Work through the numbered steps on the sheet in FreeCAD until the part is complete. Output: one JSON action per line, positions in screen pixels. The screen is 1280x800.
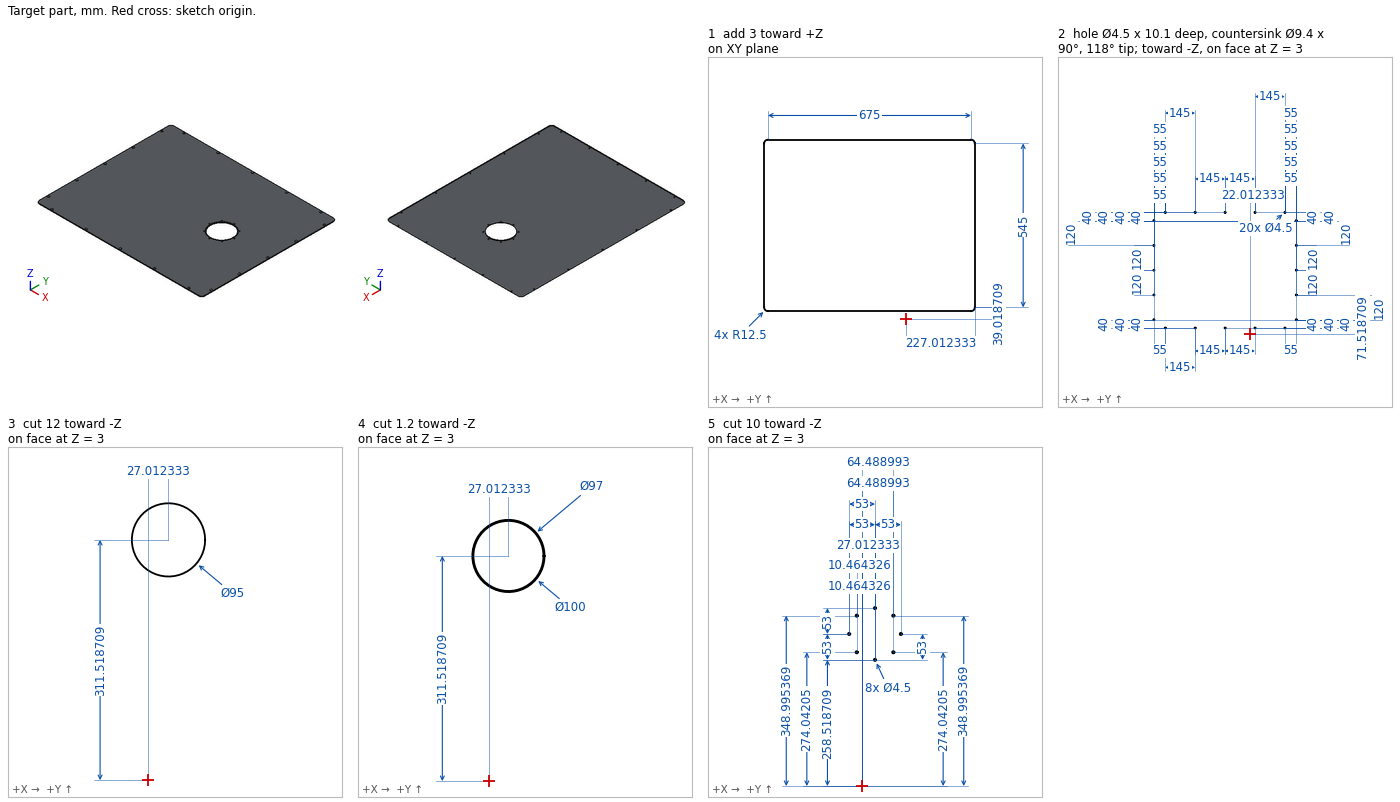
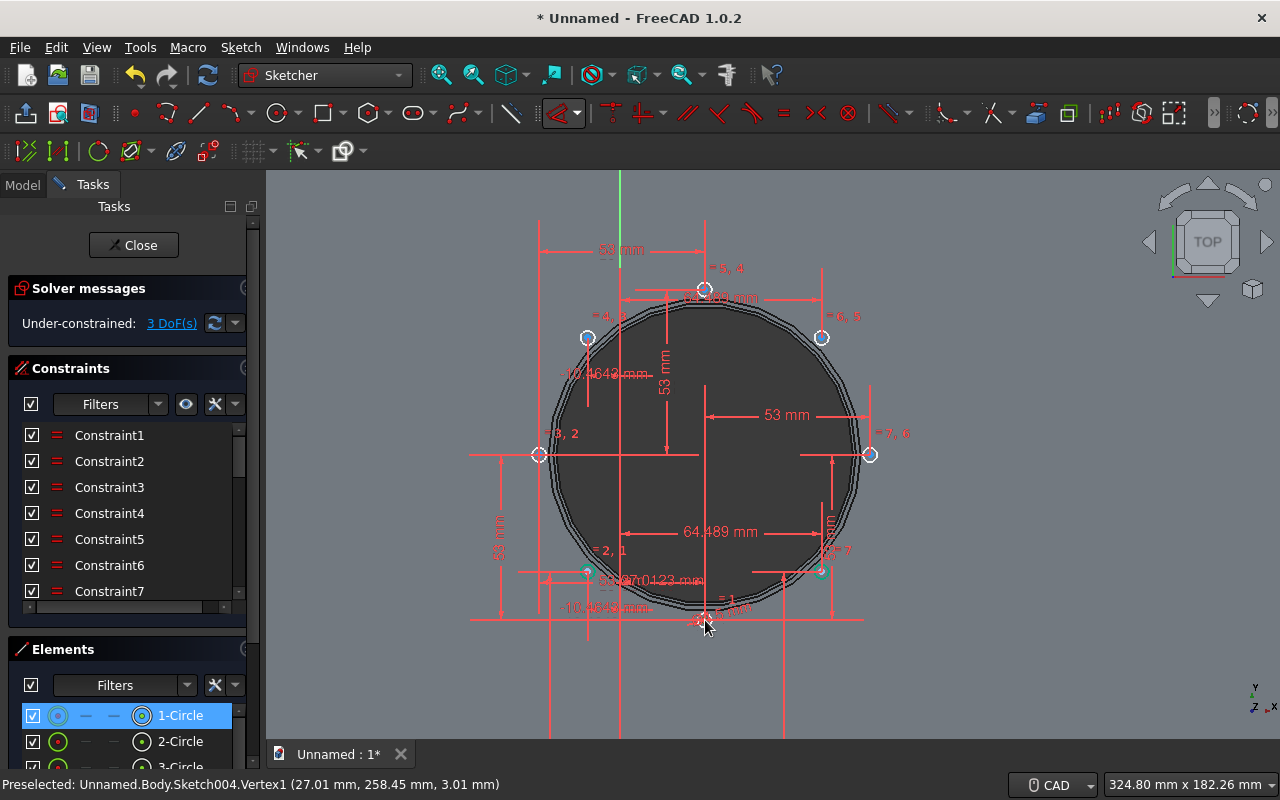
{"action": "key", "text": "i"}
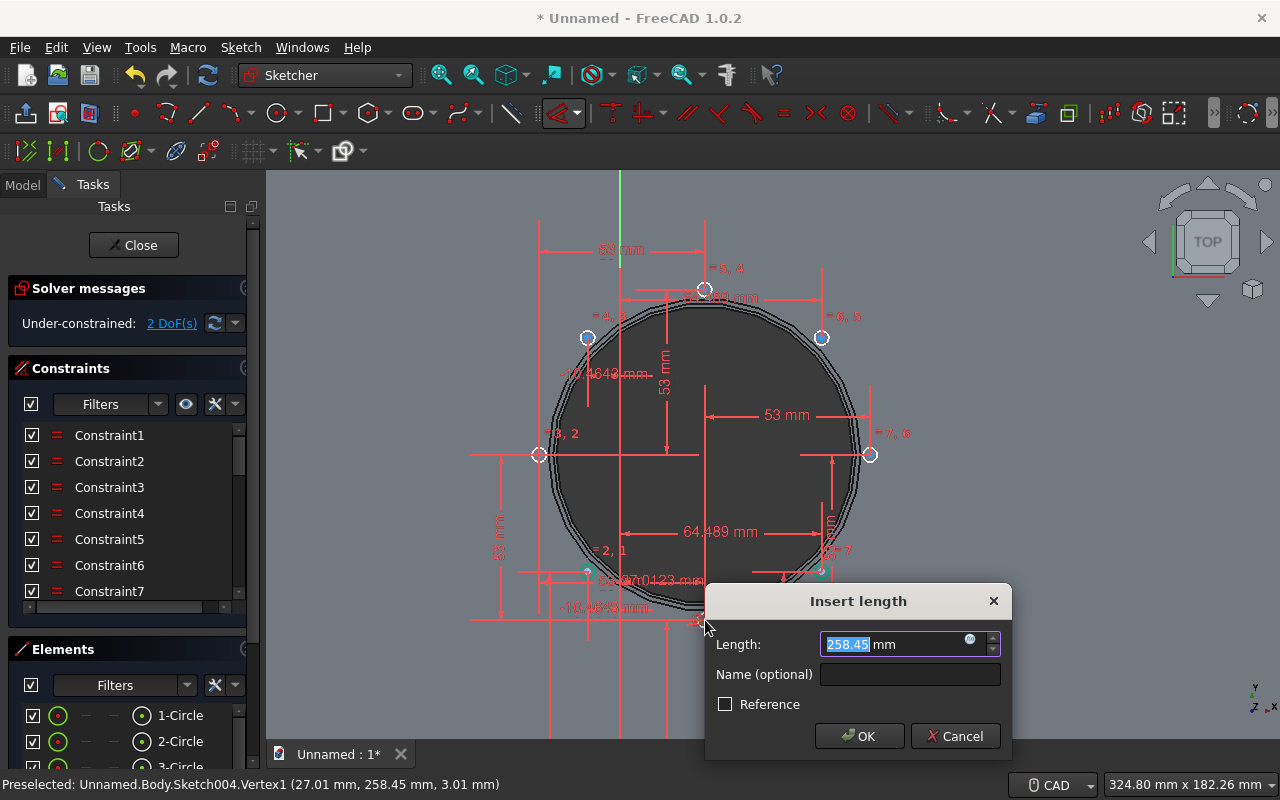
{"action": "type", "text": "258.518709"}
{"action": "key", "text": "Return"}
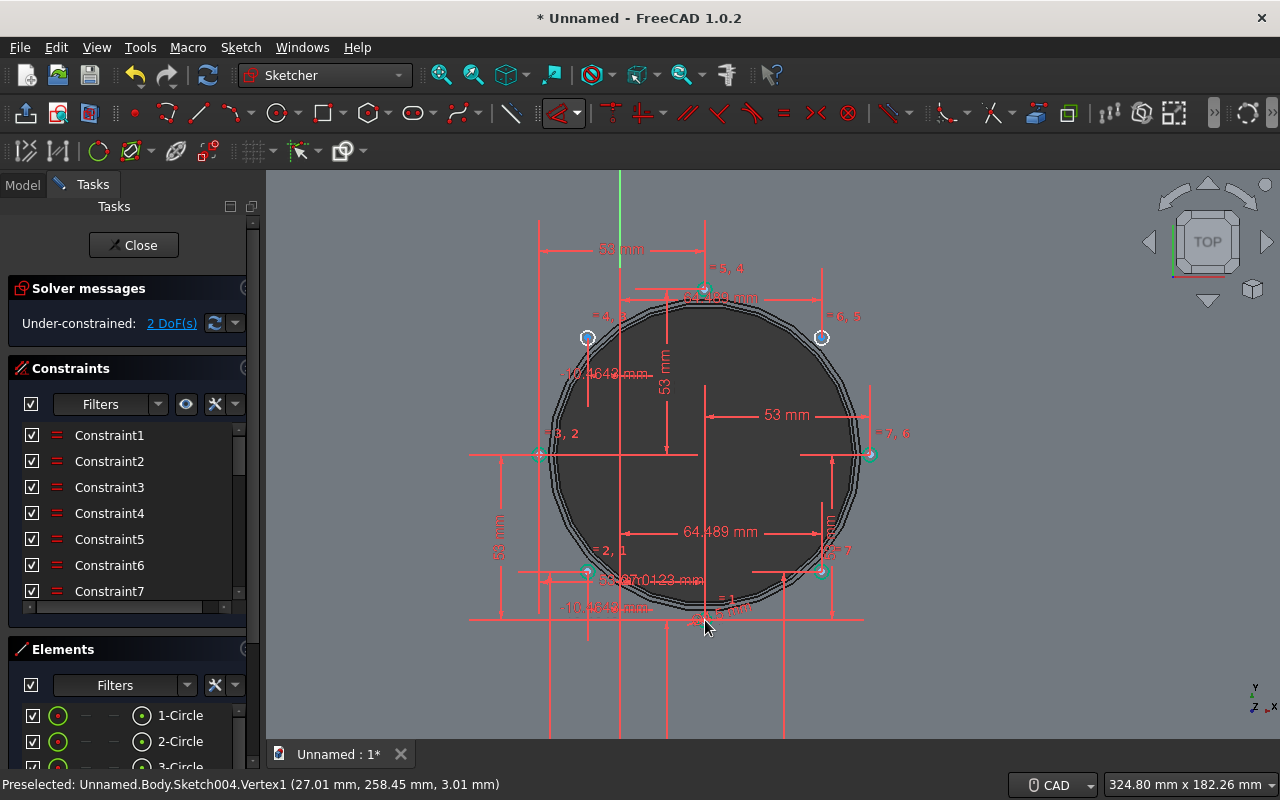
{"action": "left_click", "coordinate": [588, 338]}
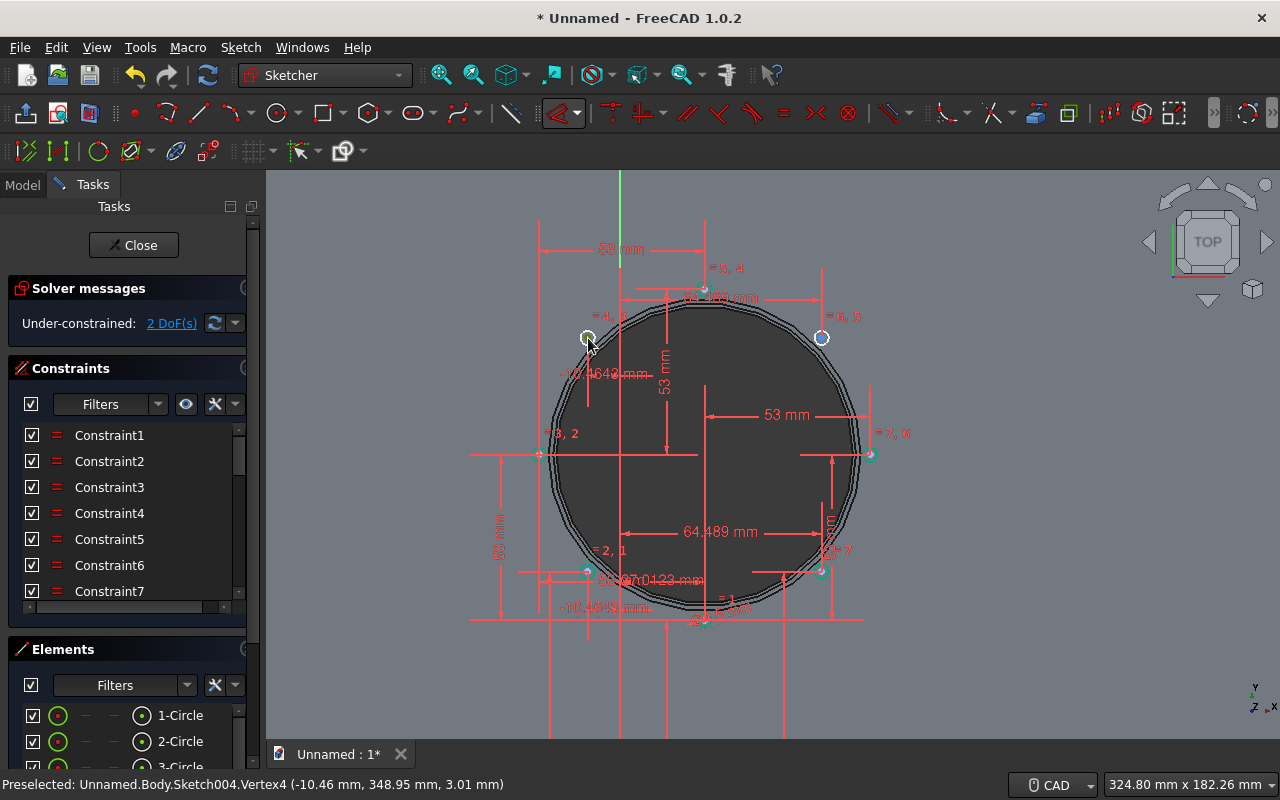
{"action": "key", "text": "i"}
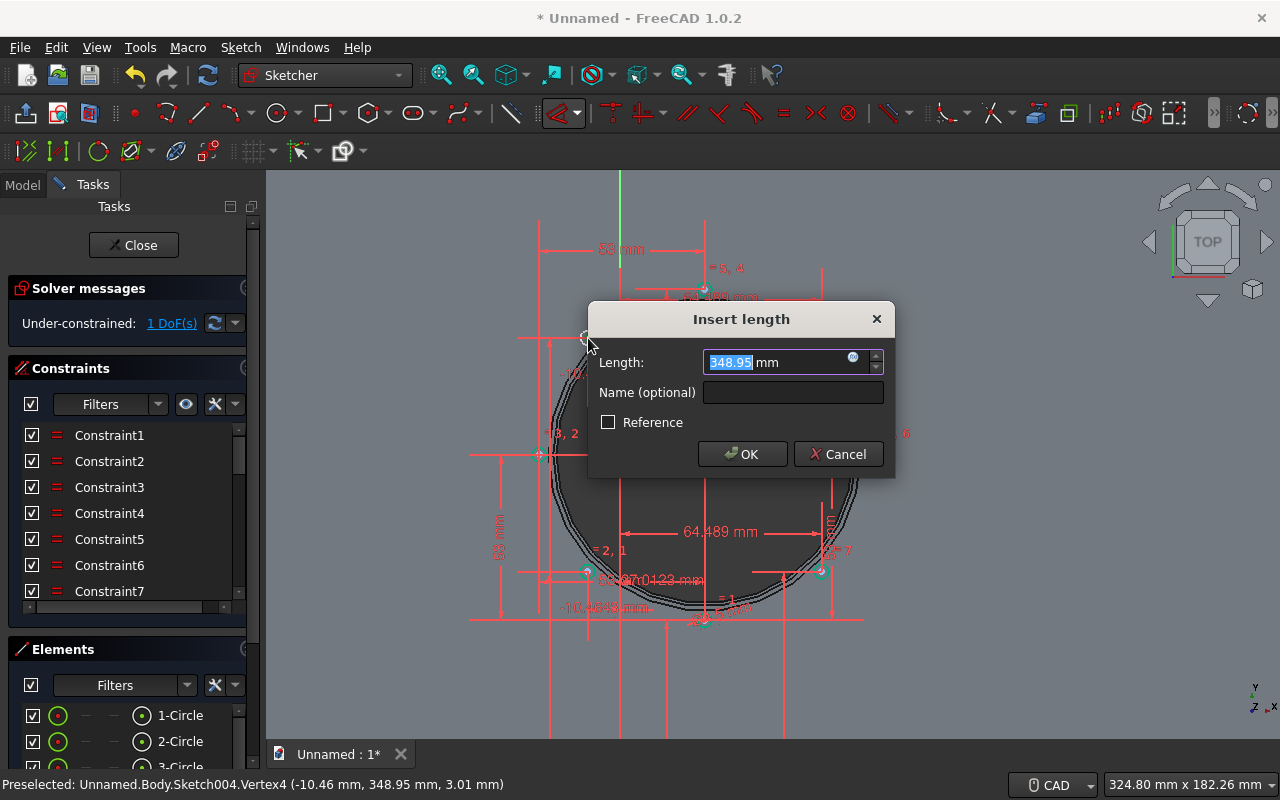
{"action": "type", "text": "348.995369"}
{"action": "key", "text": "Return"}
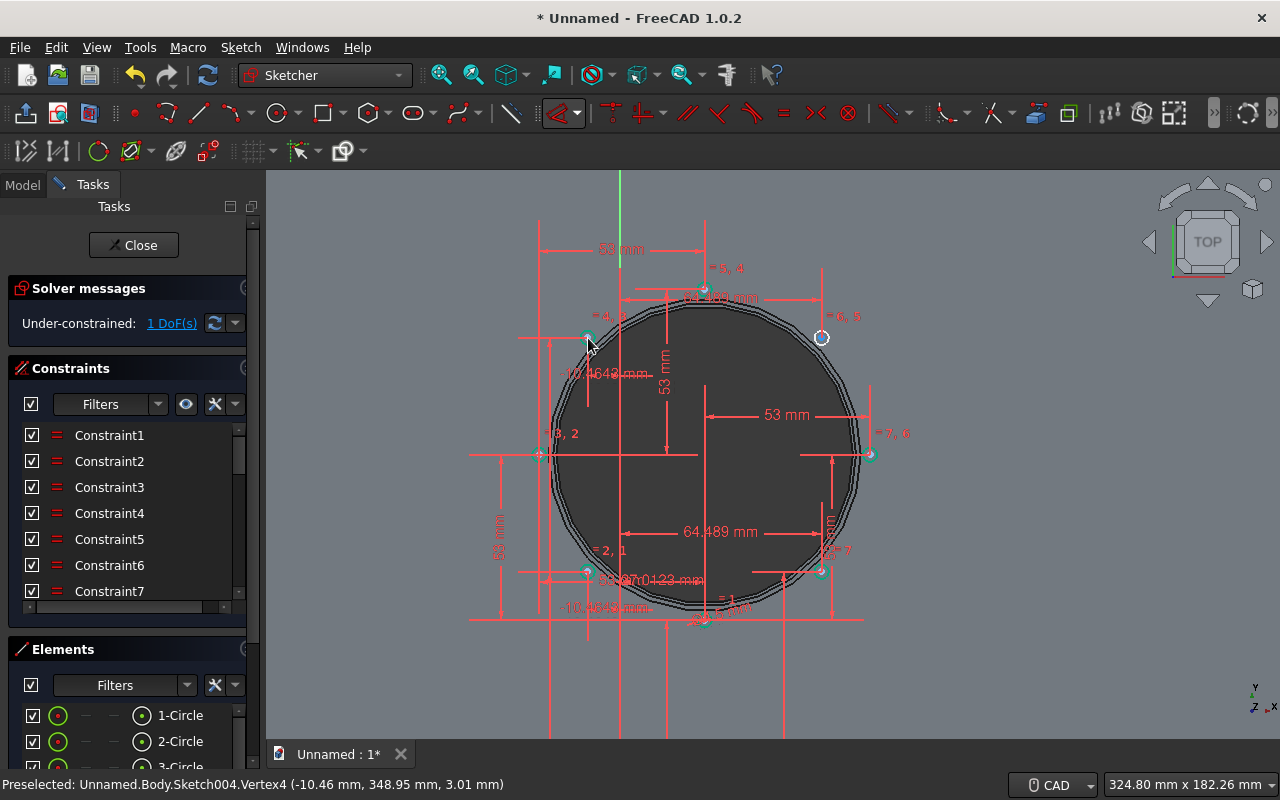
{"action": "left_click", "coordinate": [822, 338]}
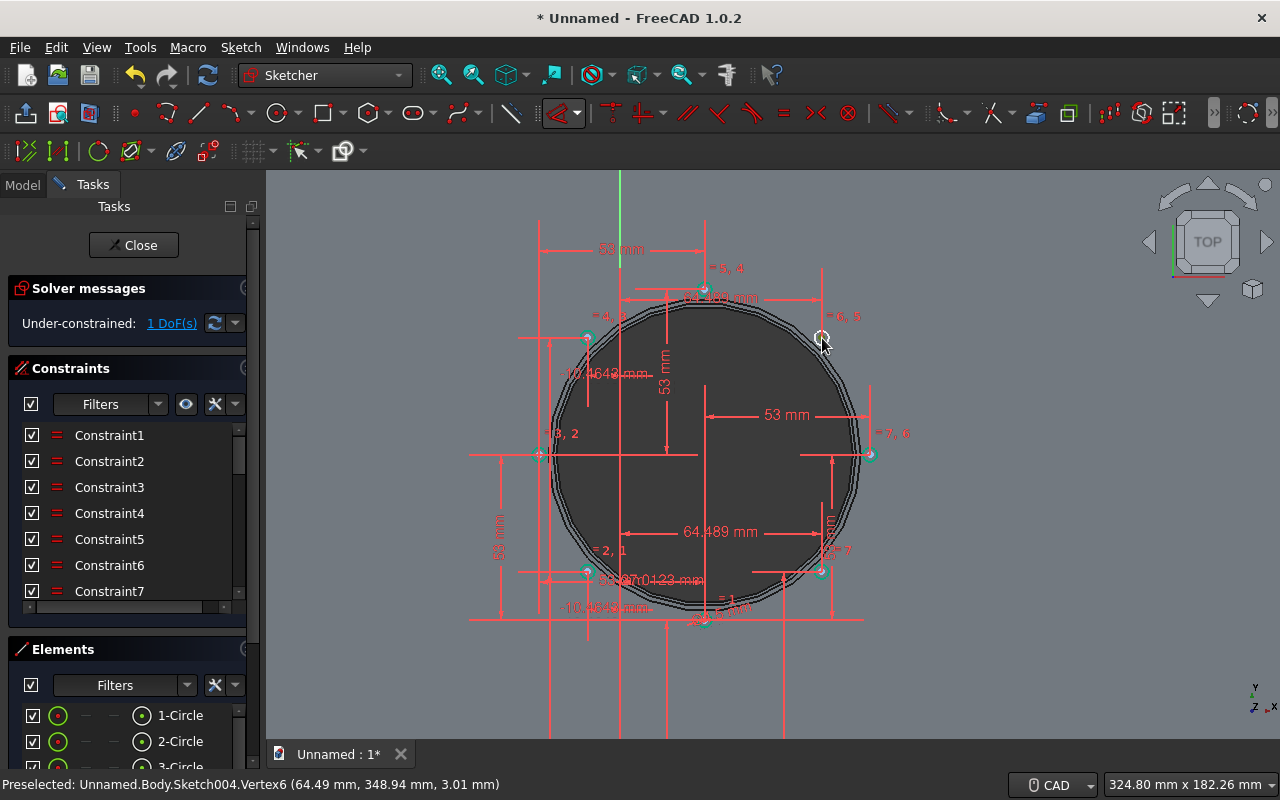
{"action": "key", "text": "i"}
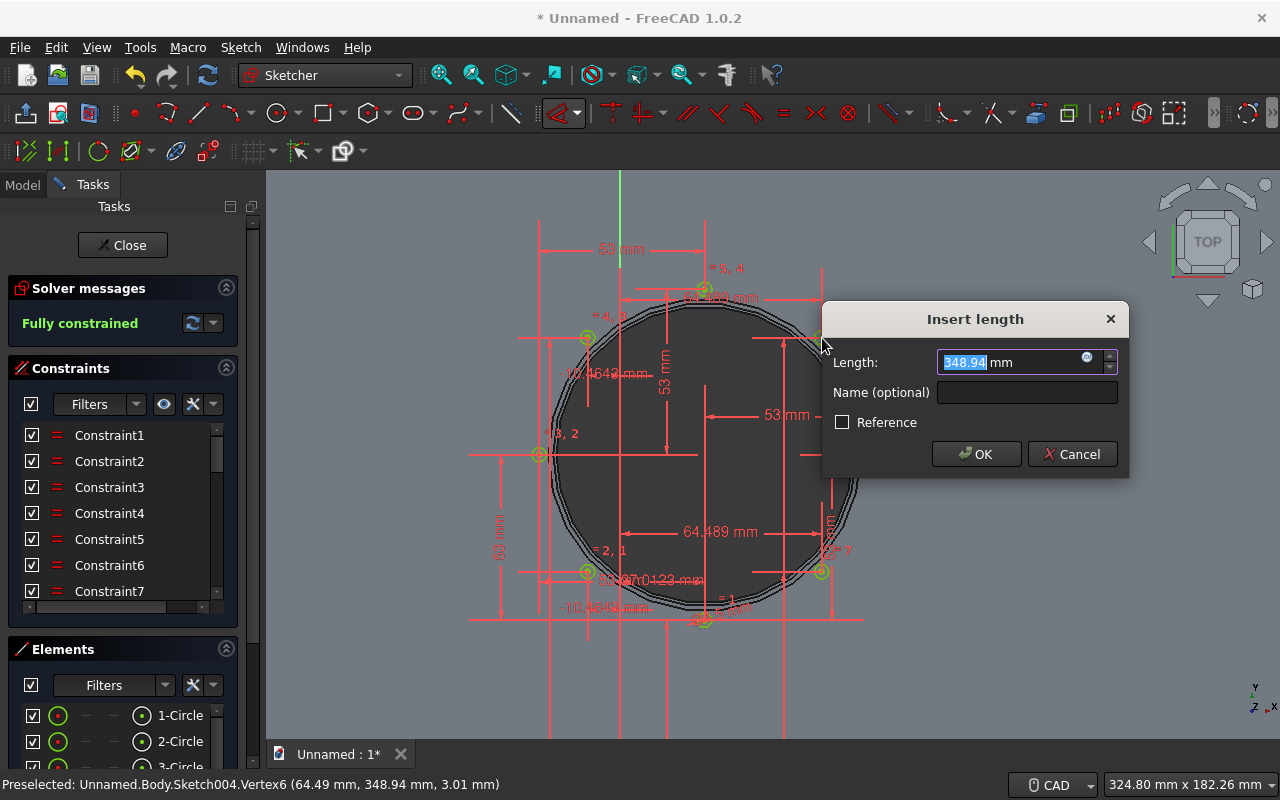
{"action": "type", "text": "348.995369"}
{"action": "key", "text": "Return"}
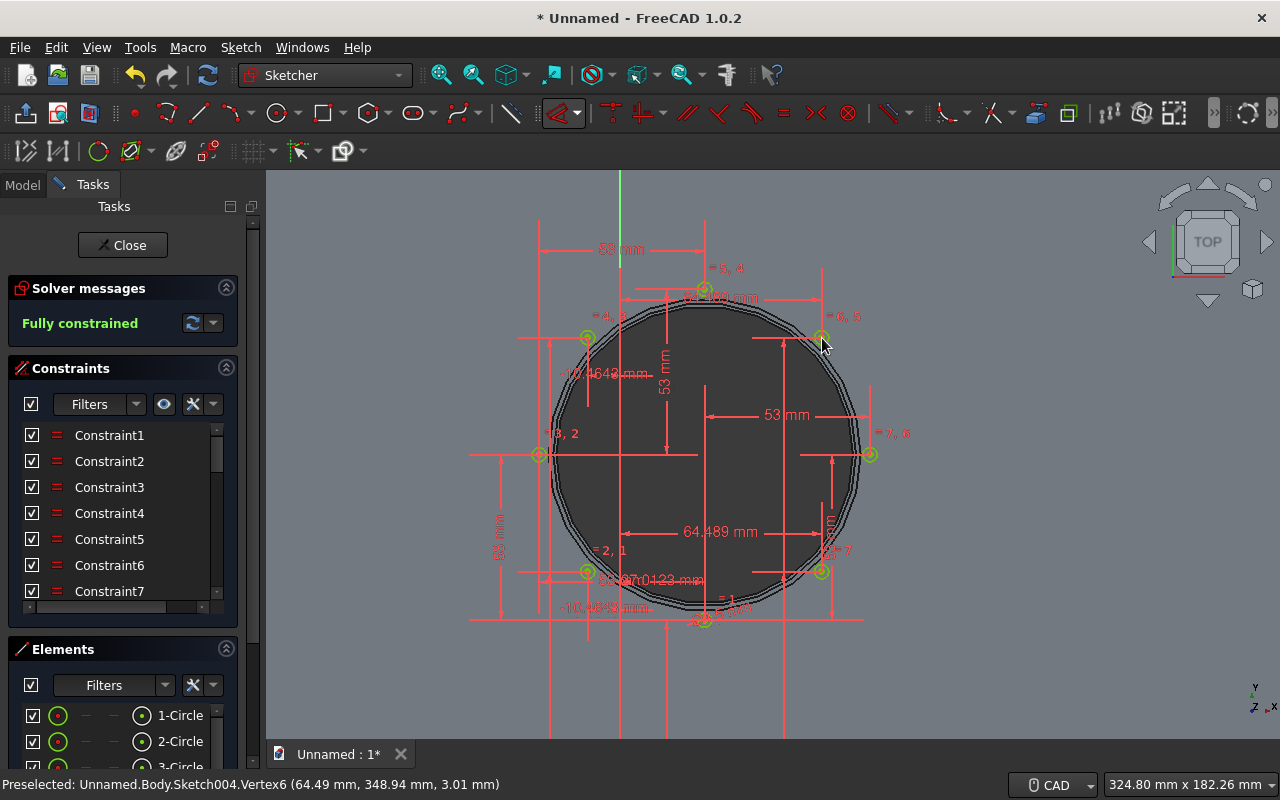
{"action": "left_click", "coordinate": [123, 245]}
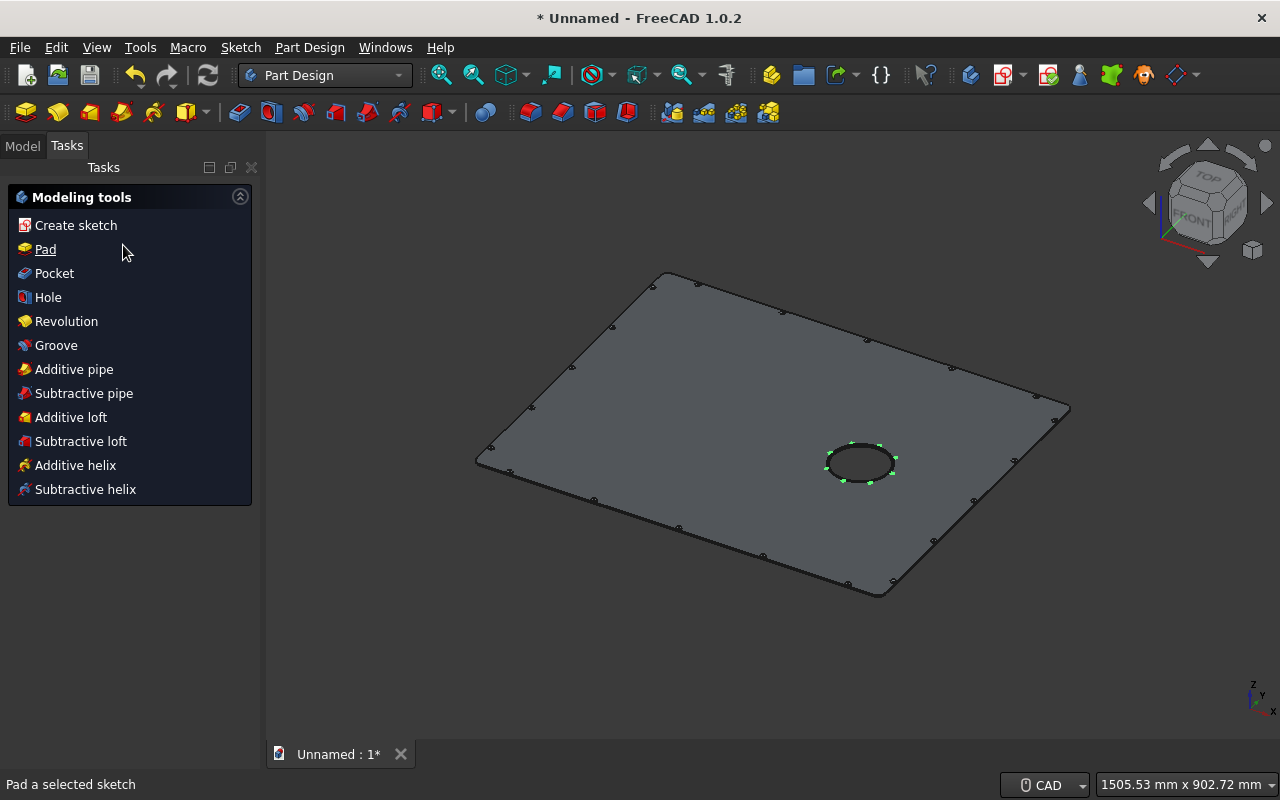
{"action": "left_click", "coordinate": [240, 112]}